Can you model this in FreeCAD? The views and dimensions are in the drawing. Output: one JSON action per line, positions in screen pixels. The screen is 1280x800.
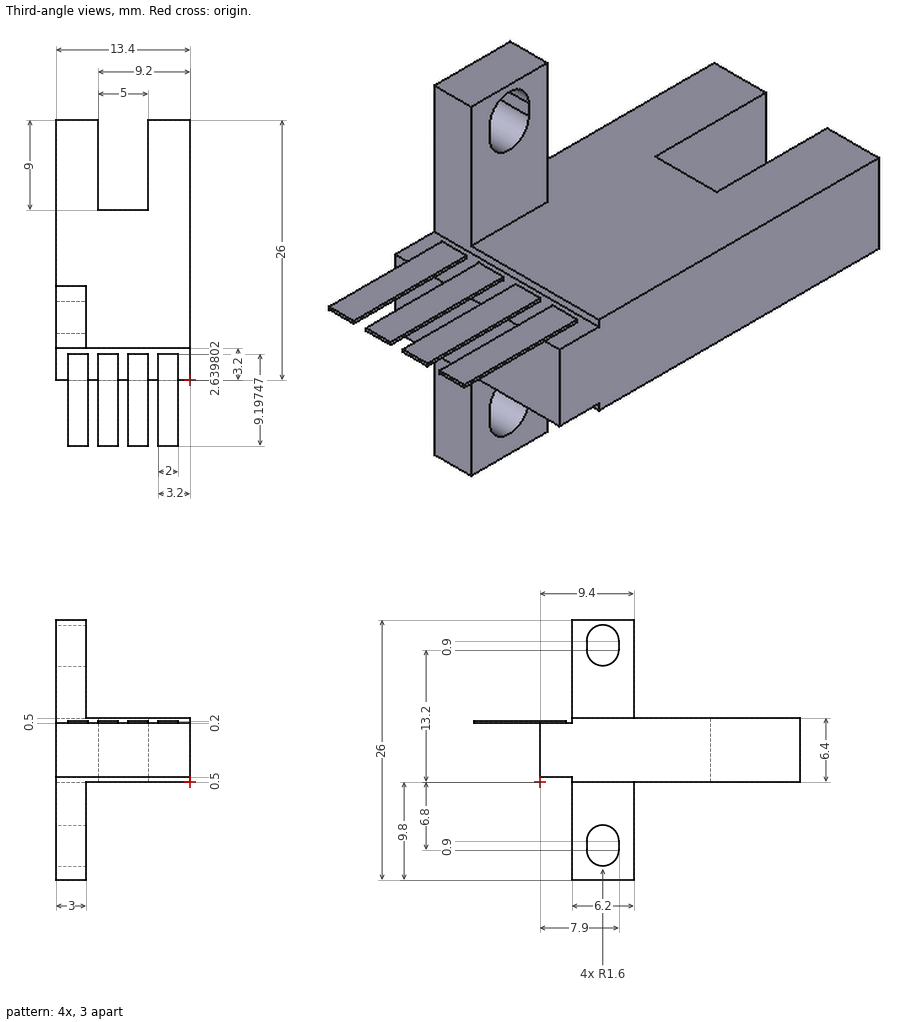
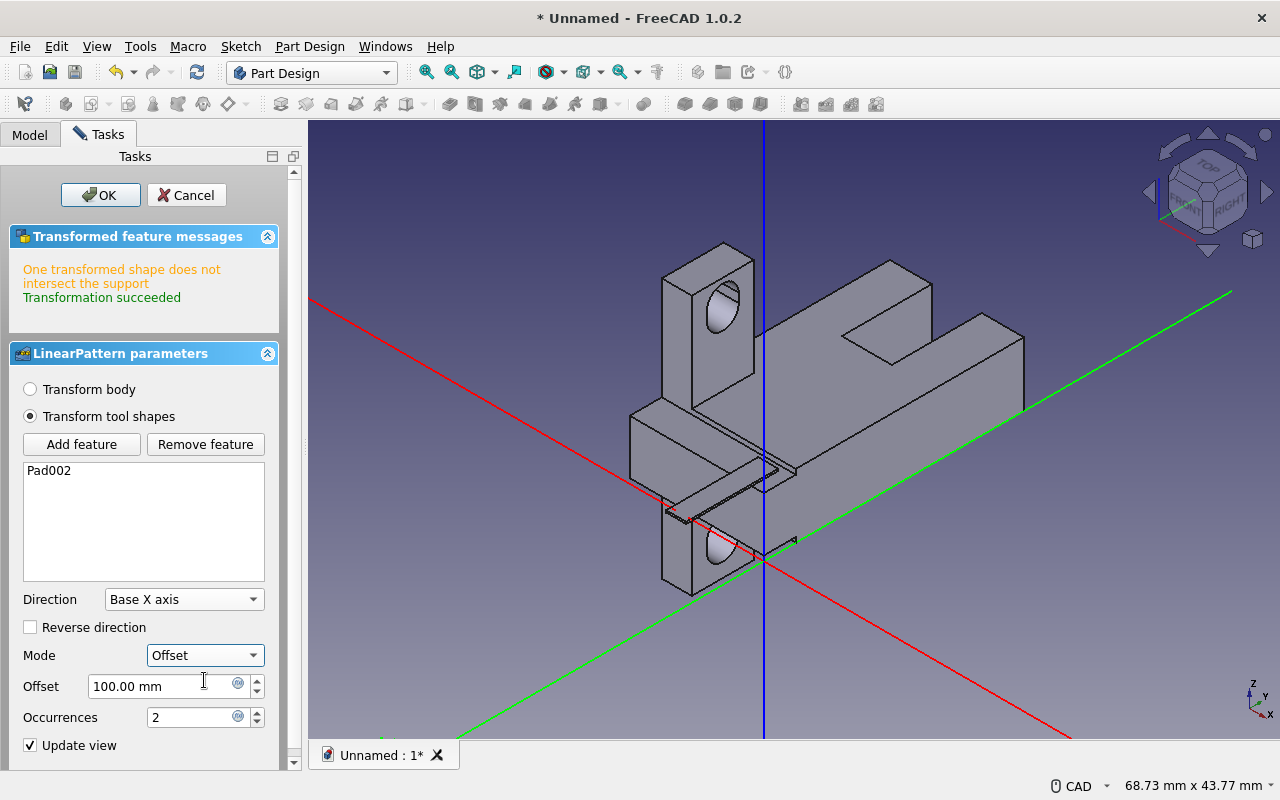
{"action": "triple_click", "coordinate": [170, 686]}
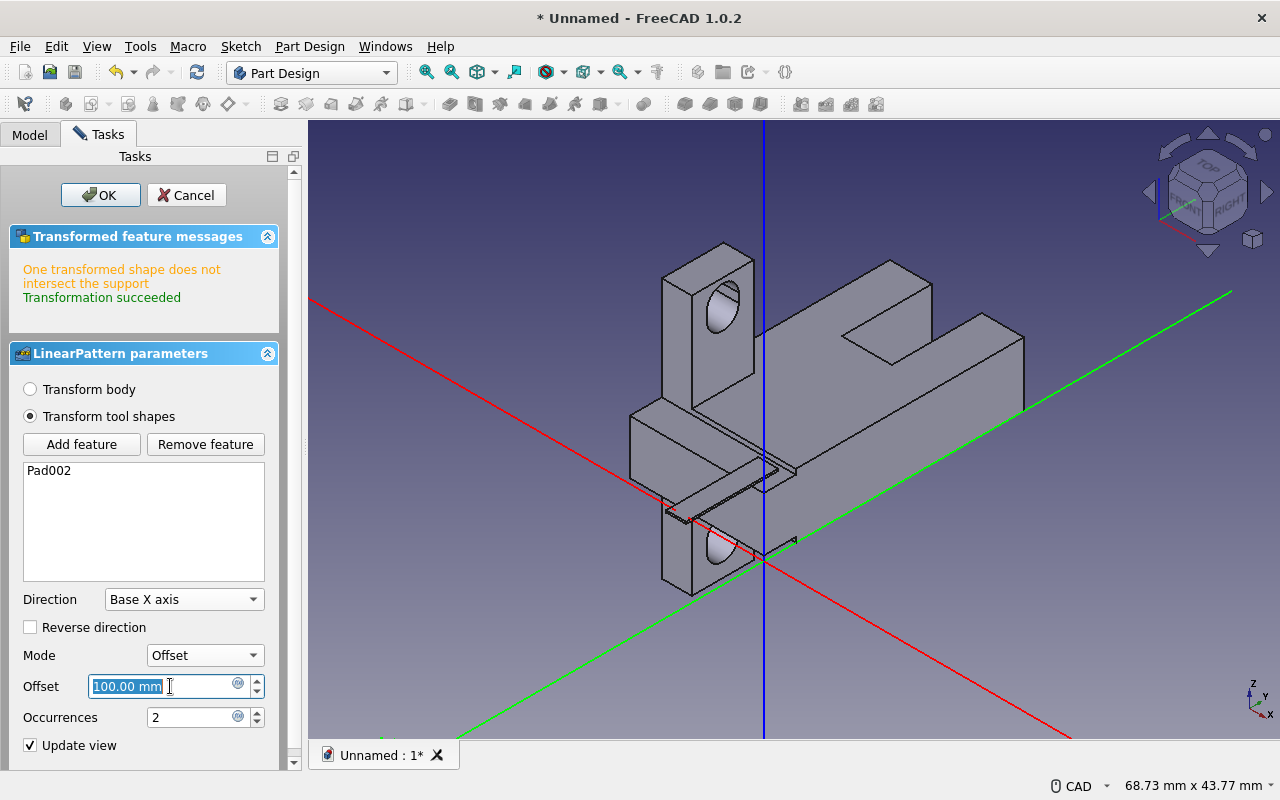
{"action": "type", "text": "3"}
{"action": "key", "text": "Tab"}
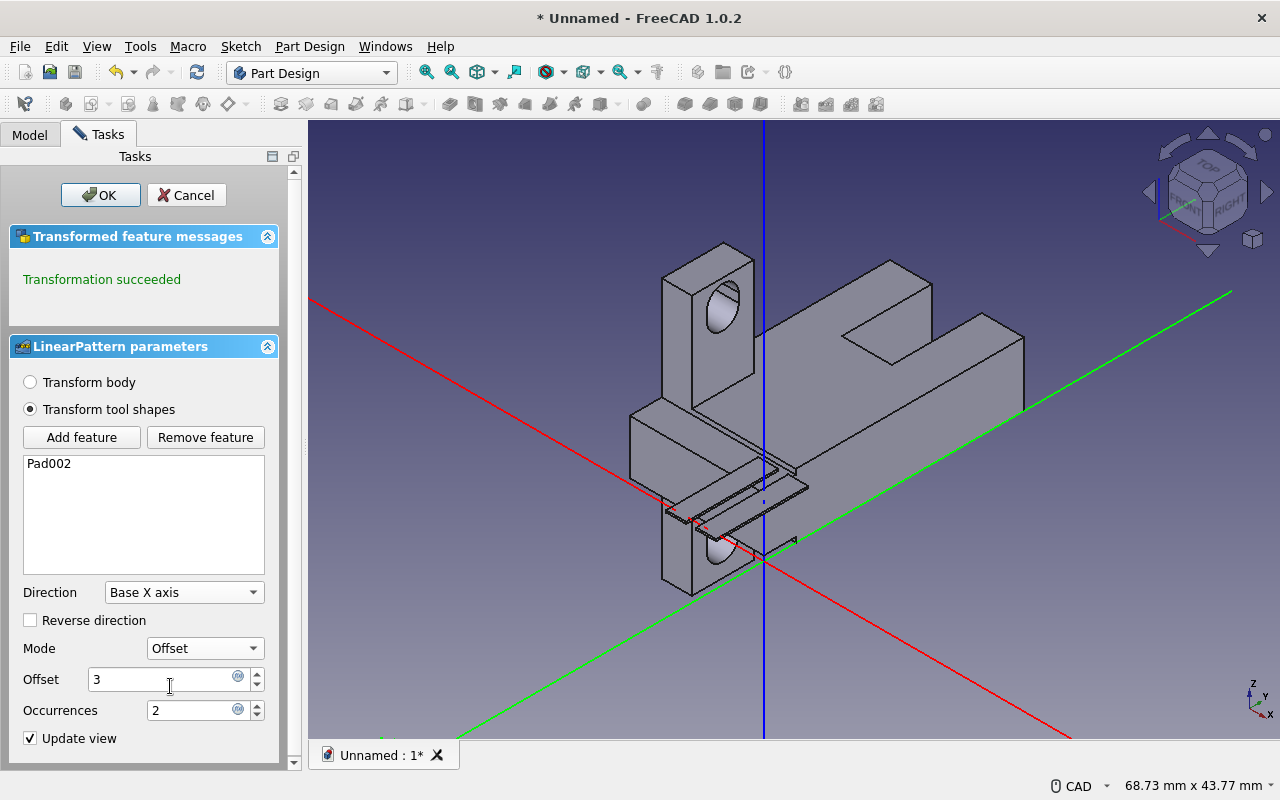
{"action": "triple_click", "coordinate": [199, 710]}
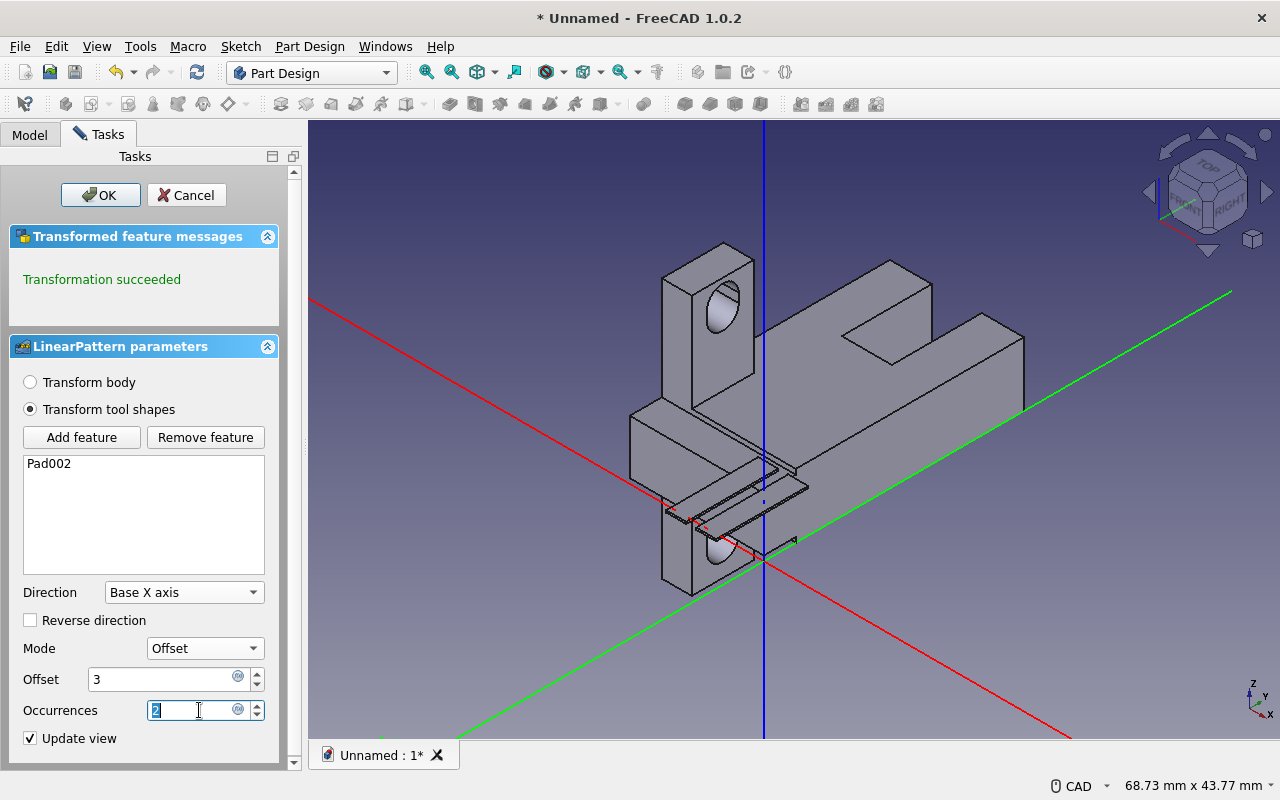
{"action": "type", "text": "4"}
{"action": "key", "text": "Tab"}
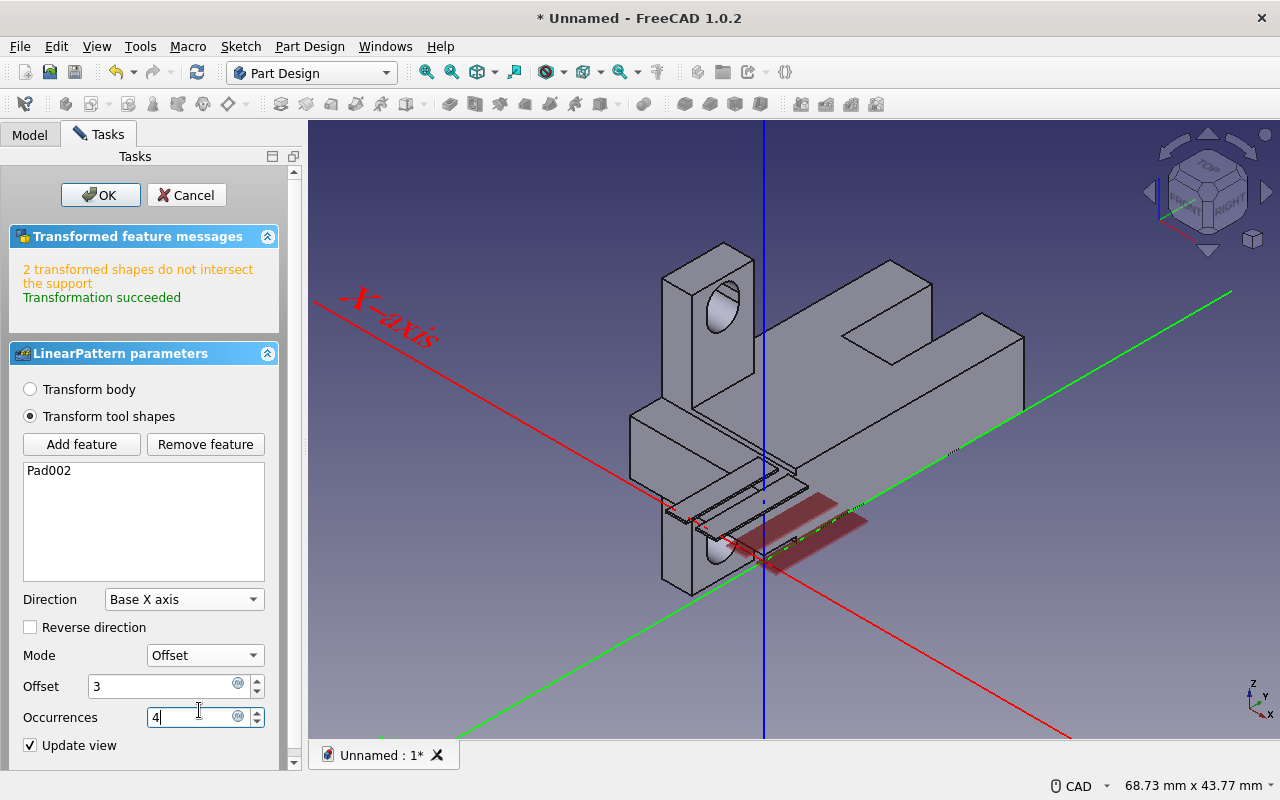
{"action": "left_click", "coordinate": [31, 627]}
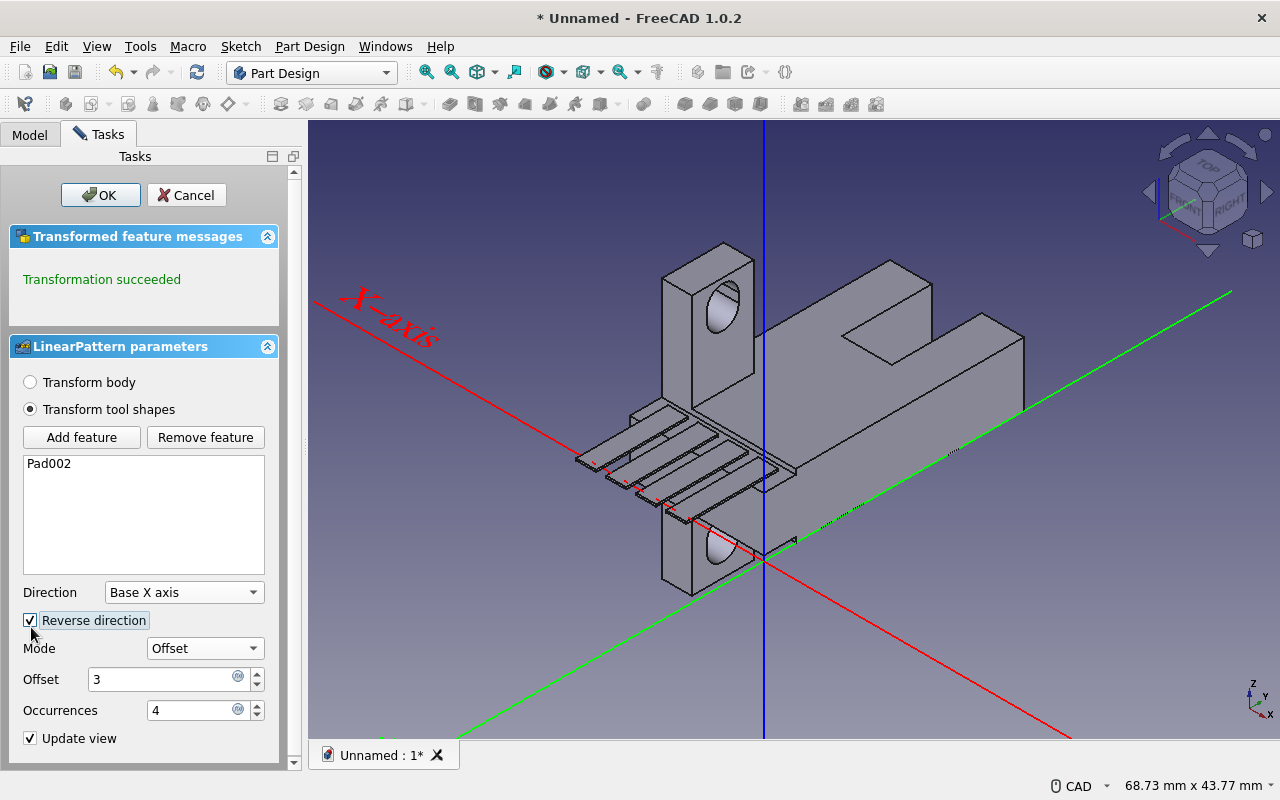
{"action": "left_click", "coordinate": [101, 195]}